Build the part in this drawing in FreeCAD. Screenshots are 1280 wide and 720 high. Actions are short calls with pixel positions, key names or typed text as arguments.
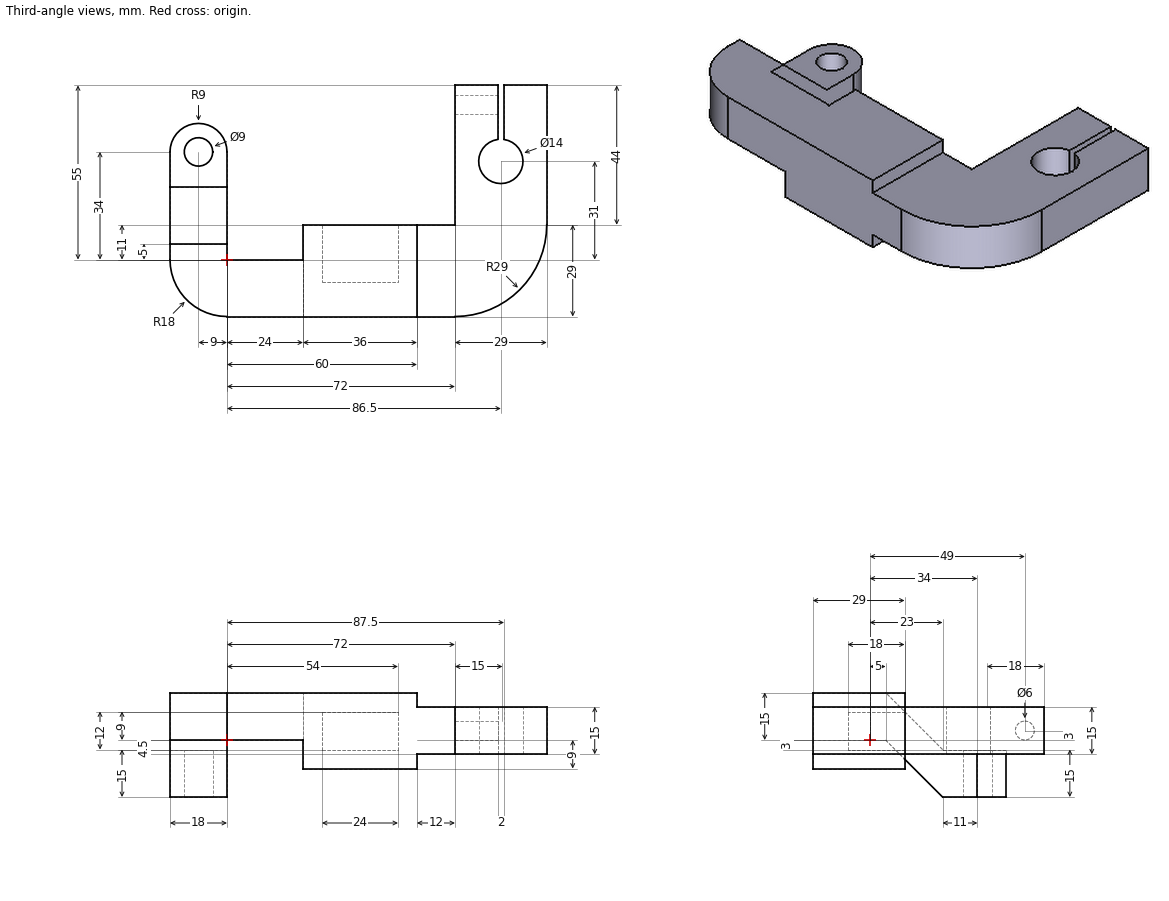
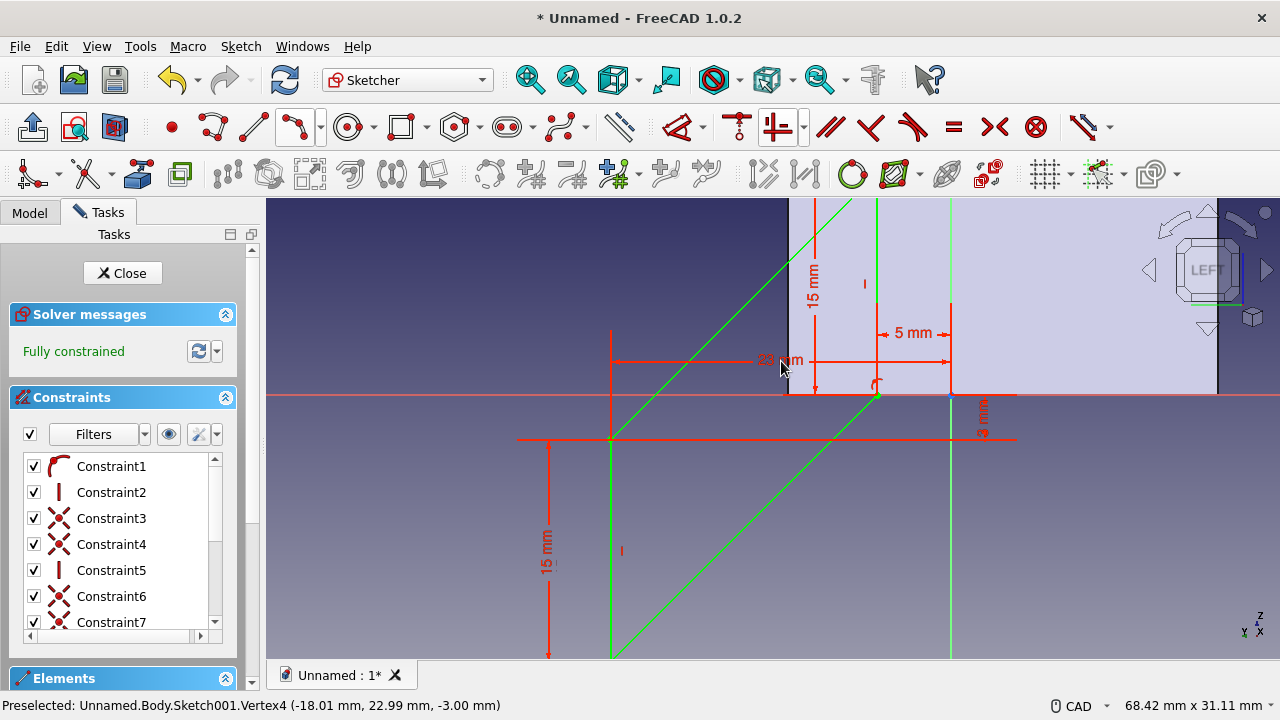
click(123, 273)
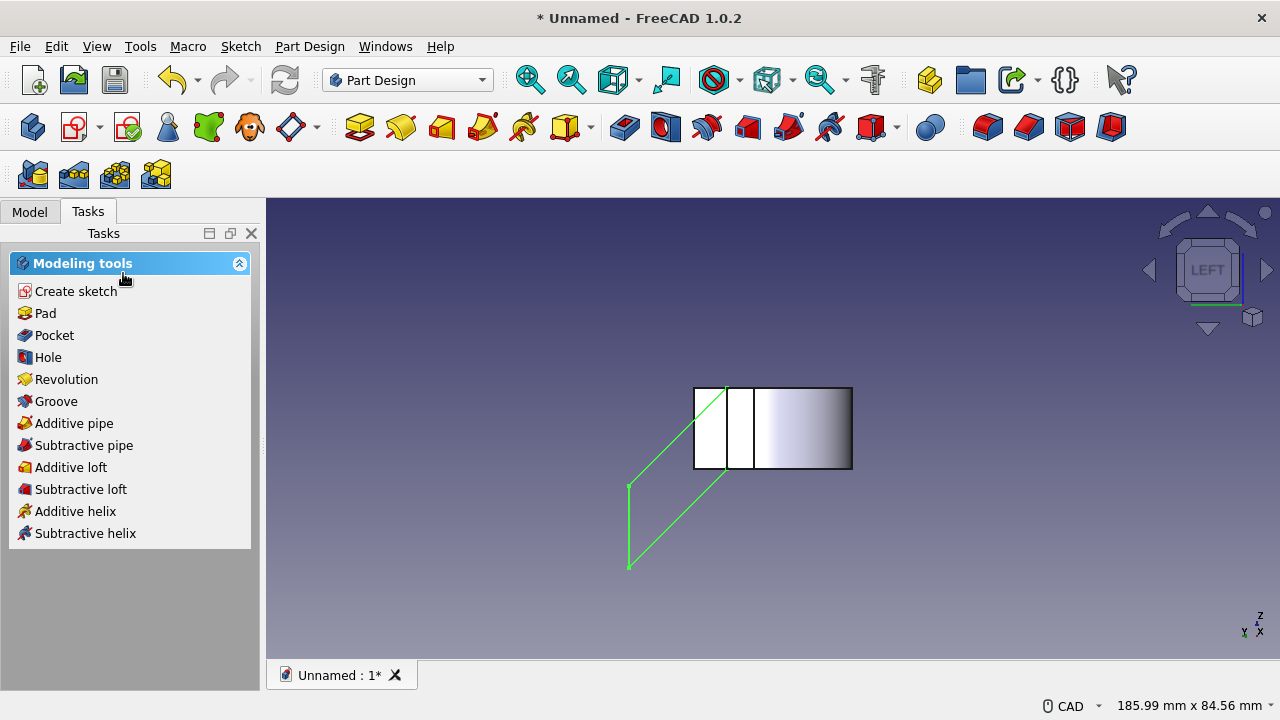
click(360, 128)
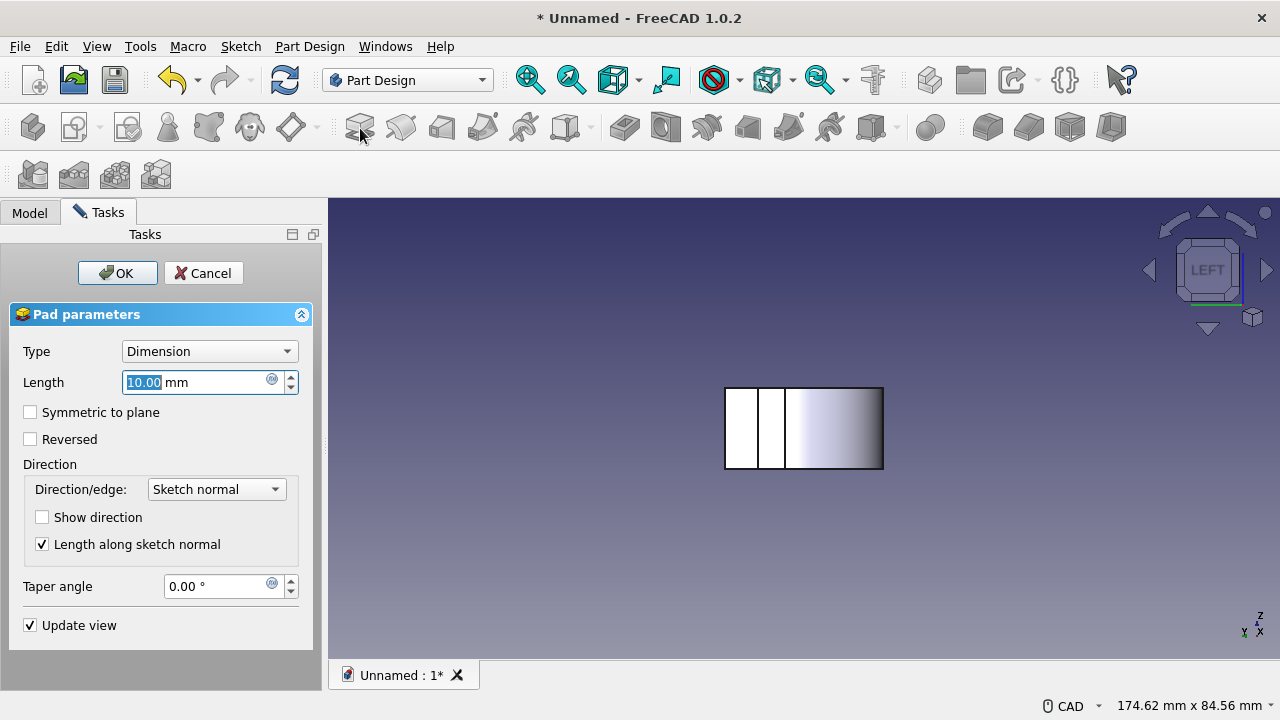
text(18)
key(Tab)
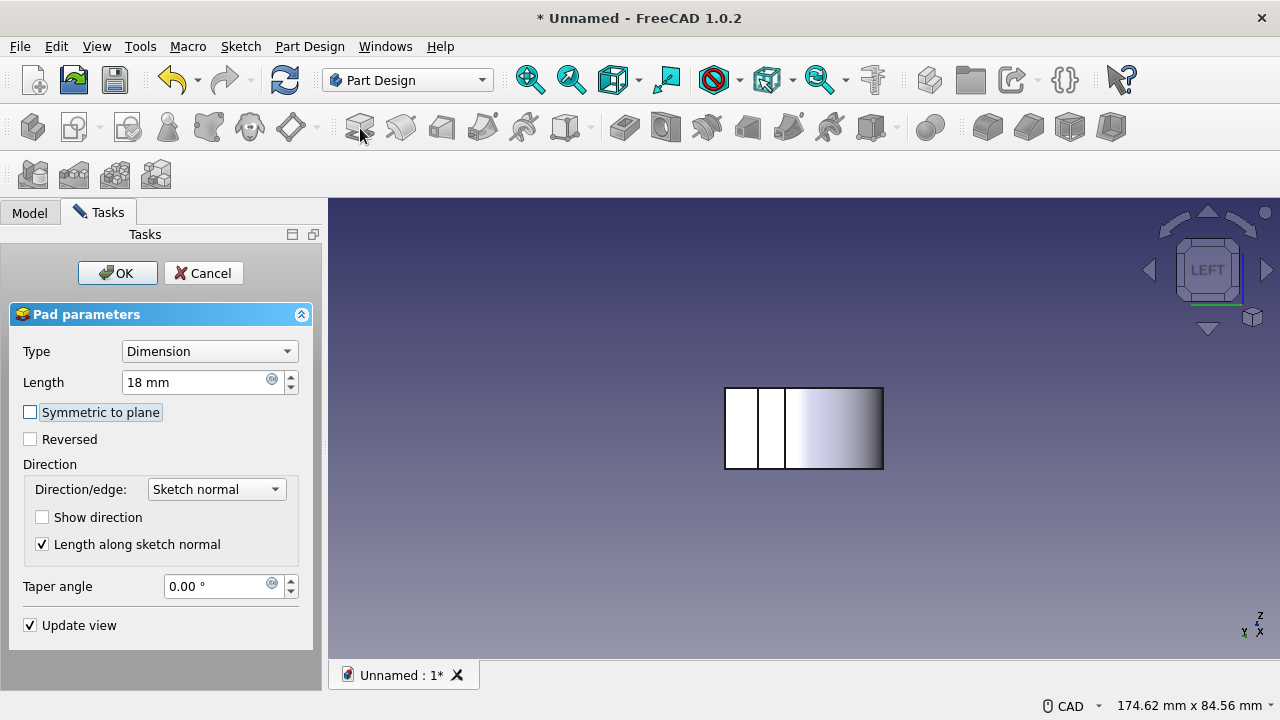
click(31, 439)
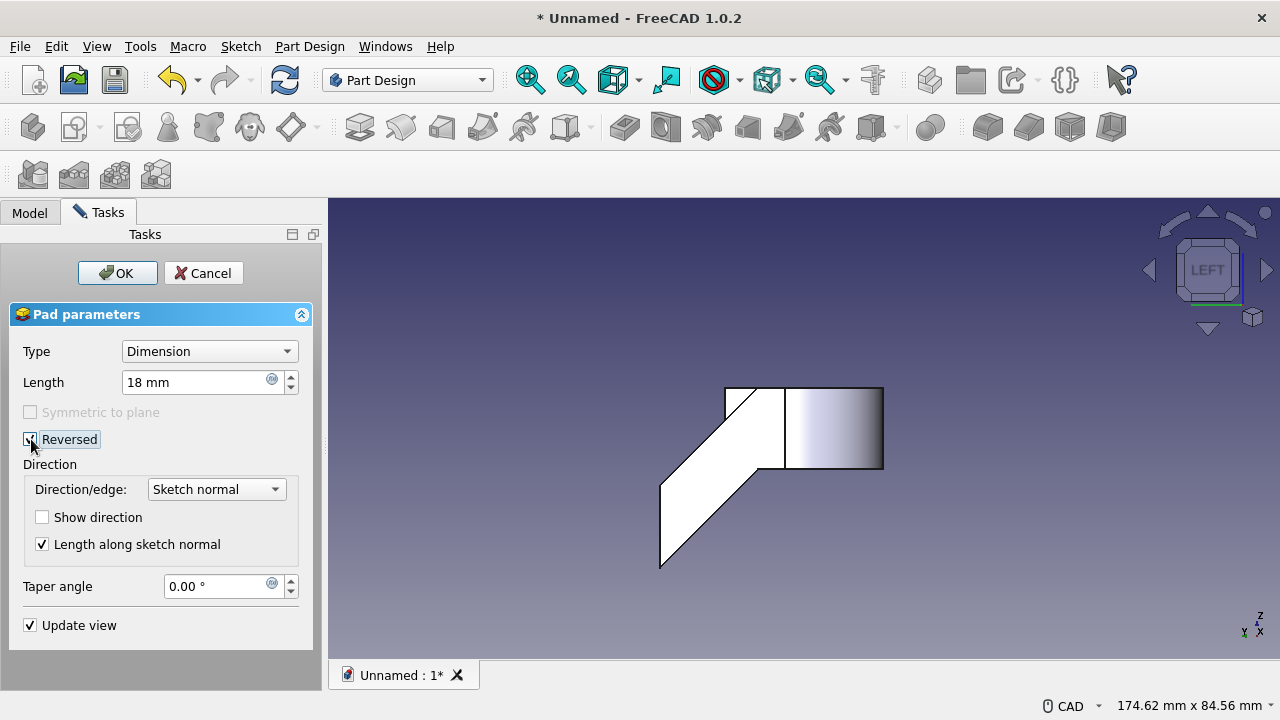
click(118, 273)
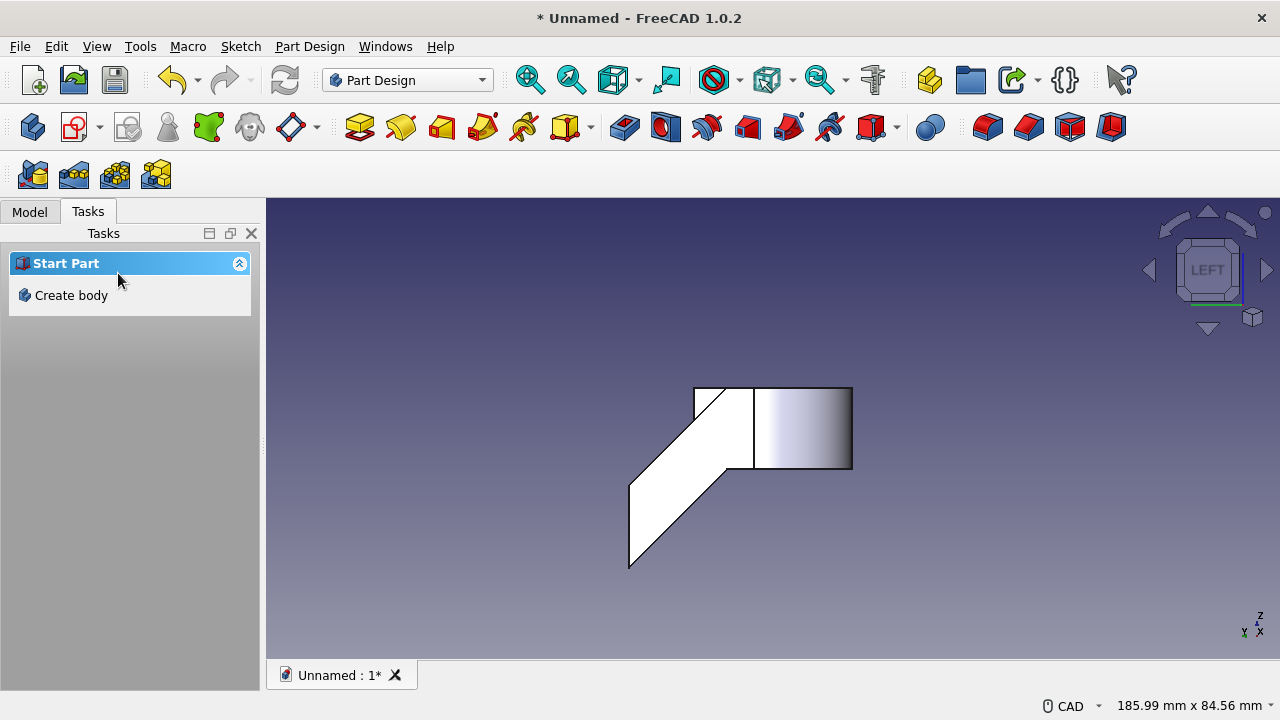
click(531, 80)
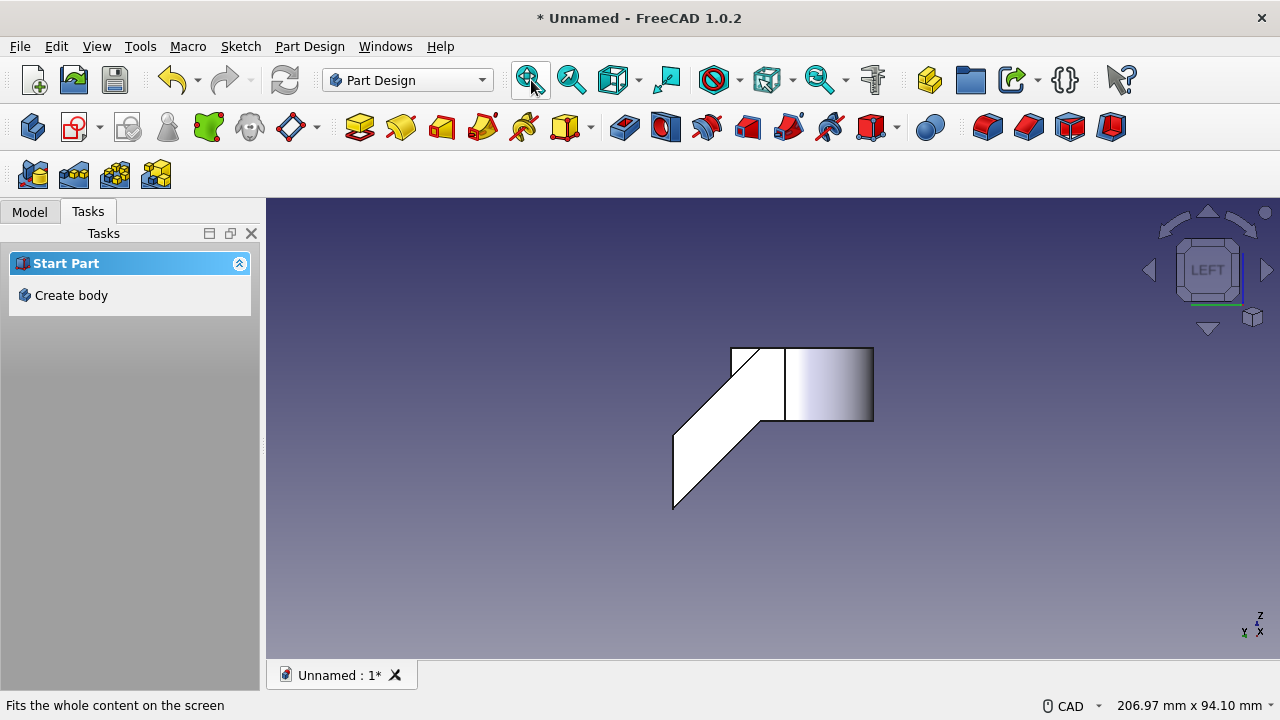
click(761, 381)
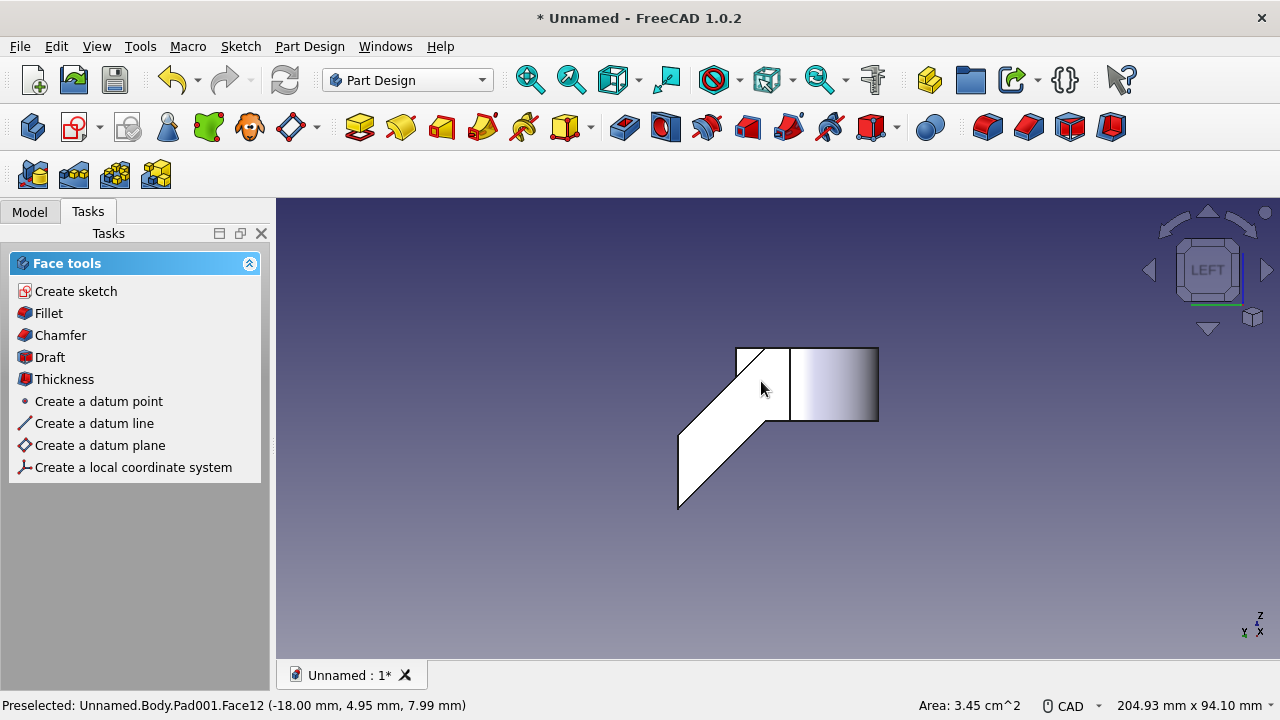
click(74, 128)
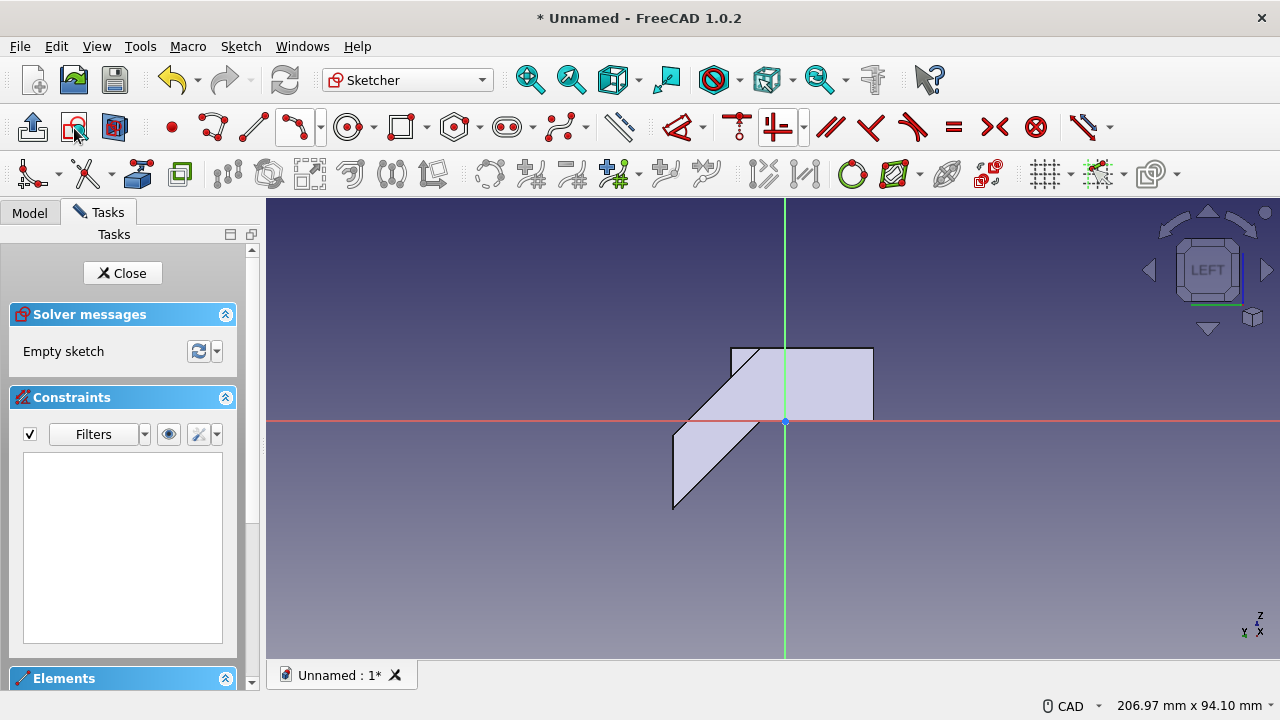
scroll(701, 481, up, 6)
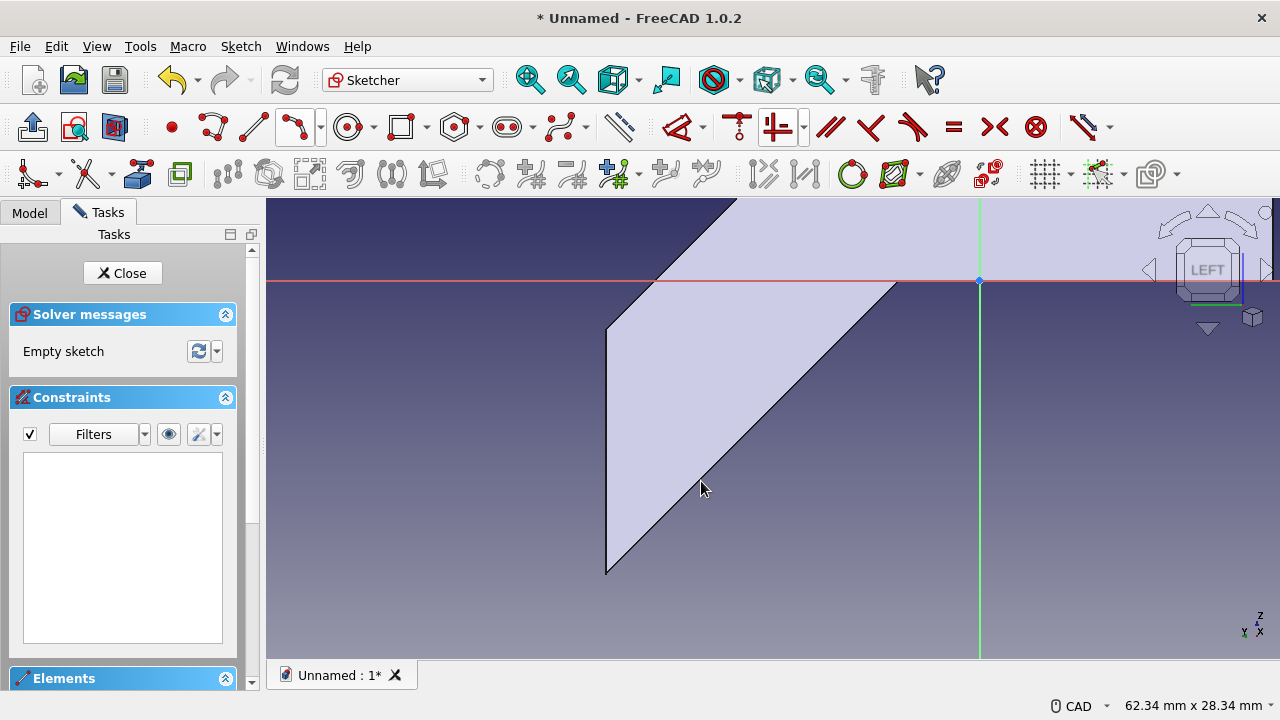
click(400, 128)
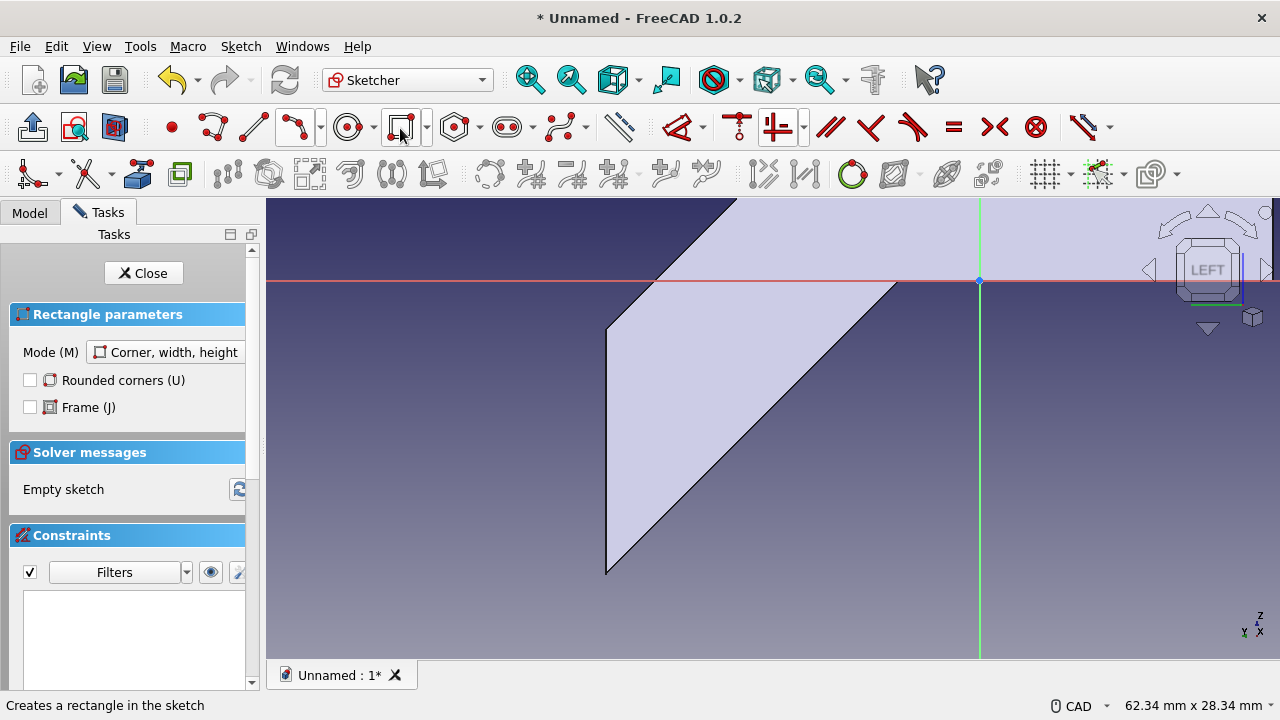
click(427, 330)
move(606, 574)